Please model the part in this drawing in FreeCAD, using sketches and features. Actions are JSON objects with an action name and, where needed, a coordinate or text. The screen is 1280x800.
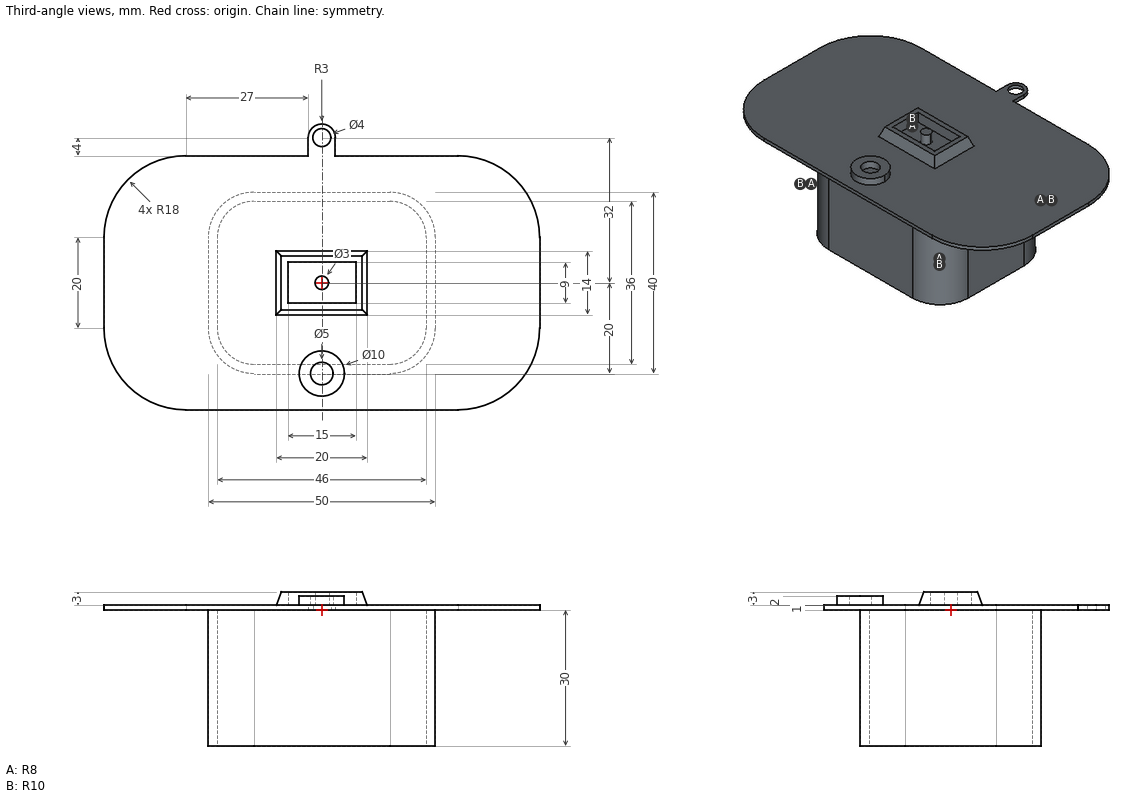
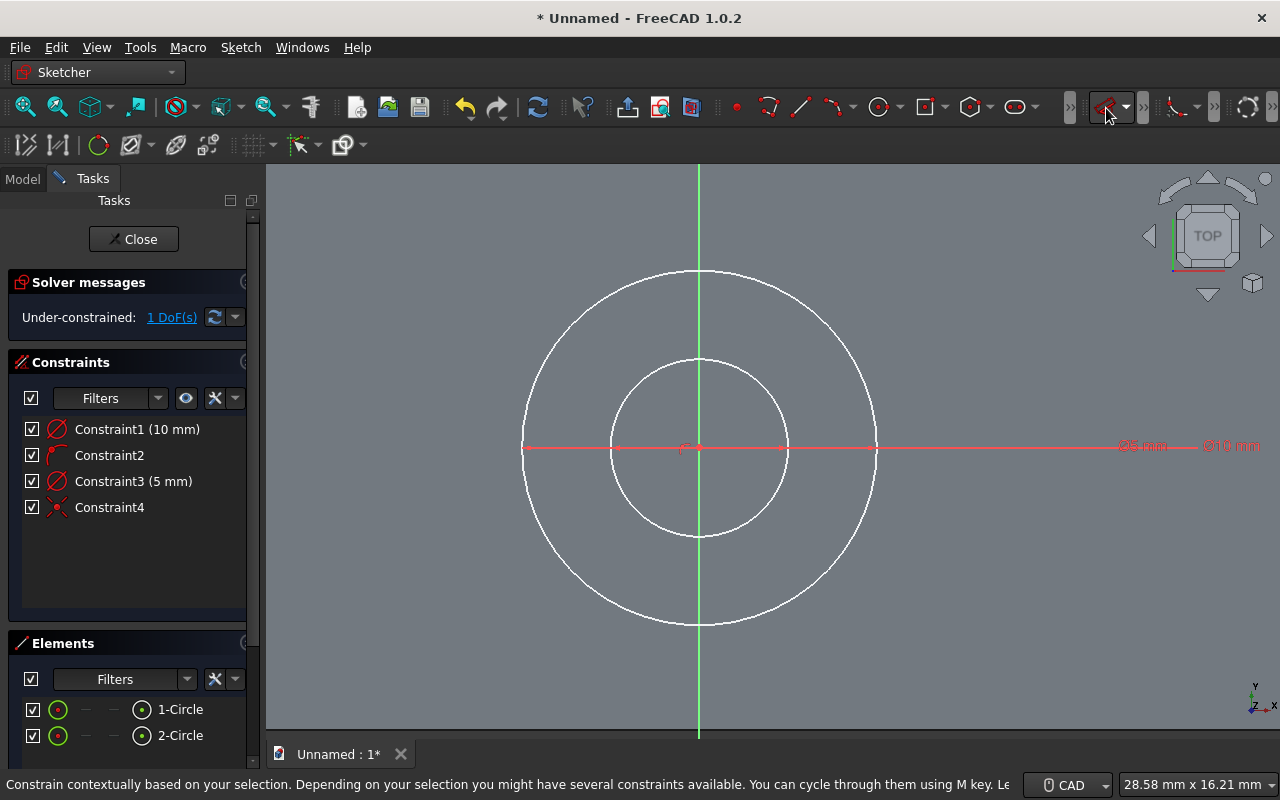
{"action": "left_click", "coordinate": [699, 448]}
{"action": "left_click", "coordinate": [733, 320]}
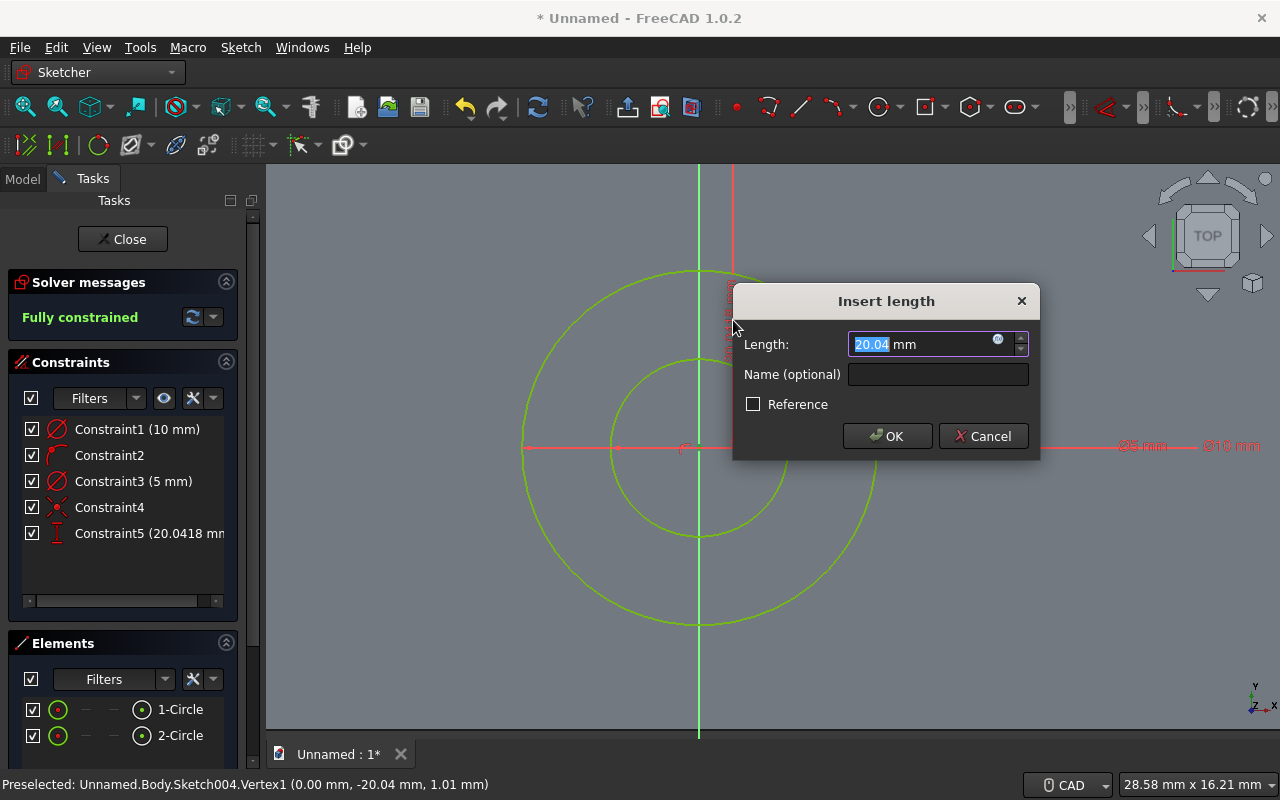
{"action": "type", "text": "20"}
{"action": "key", "text": "Return"}
{"action": "key", "text": "Escape"}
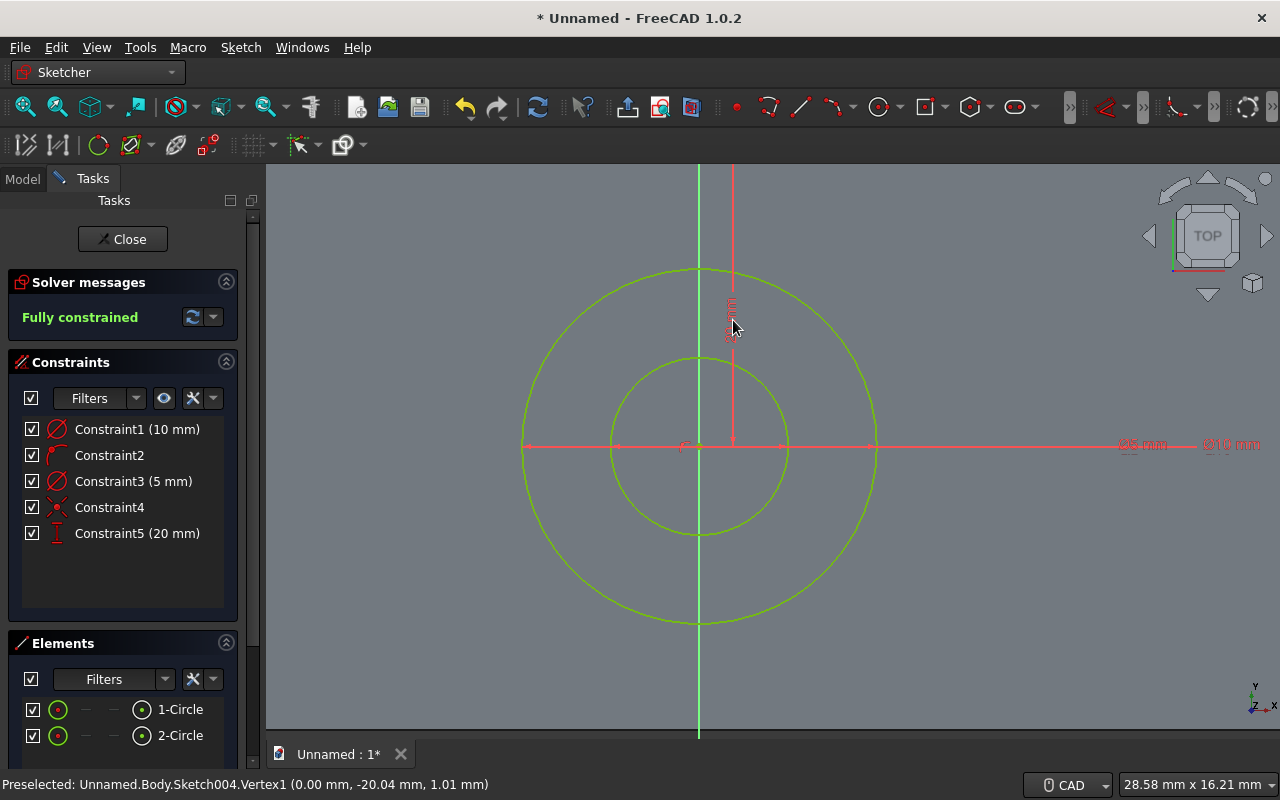
{"action": "left_click", "coordinate": [123, 239]}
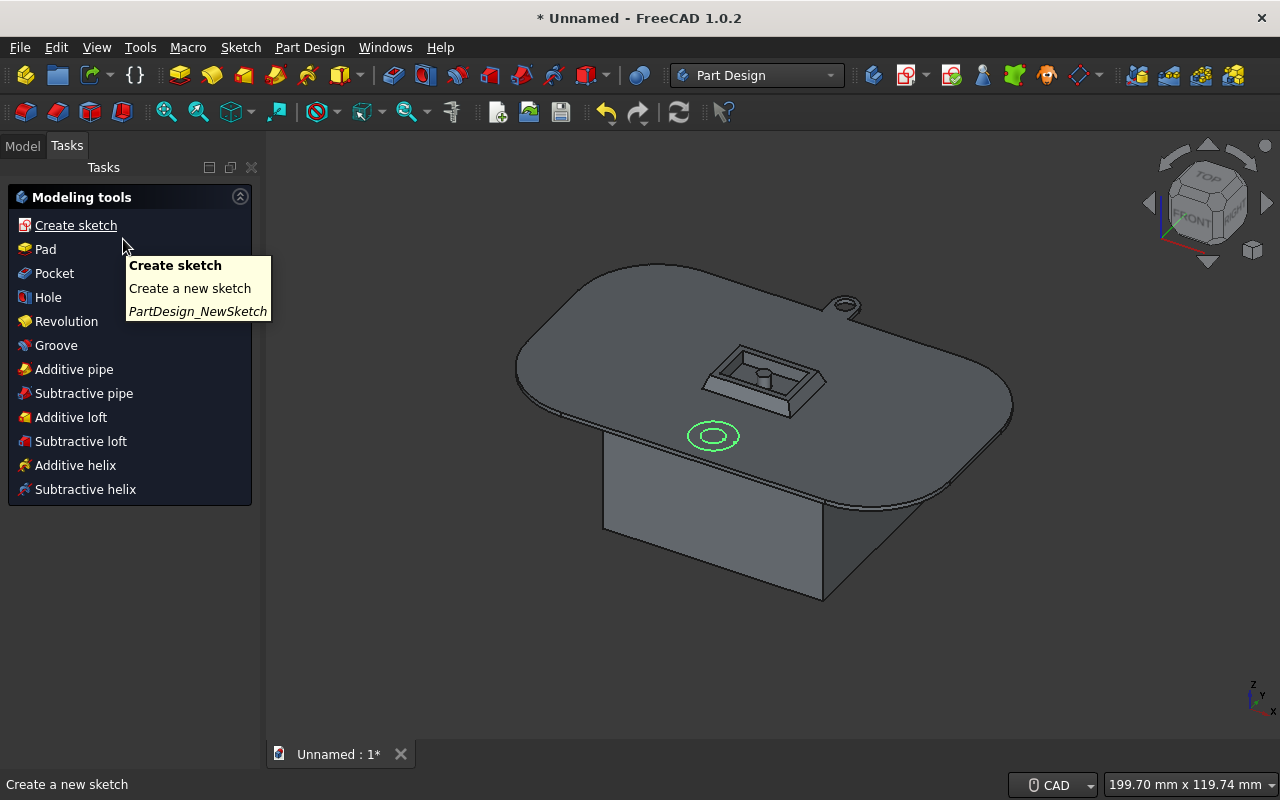
{"action": "left_click", "coordinate": [180, 76]}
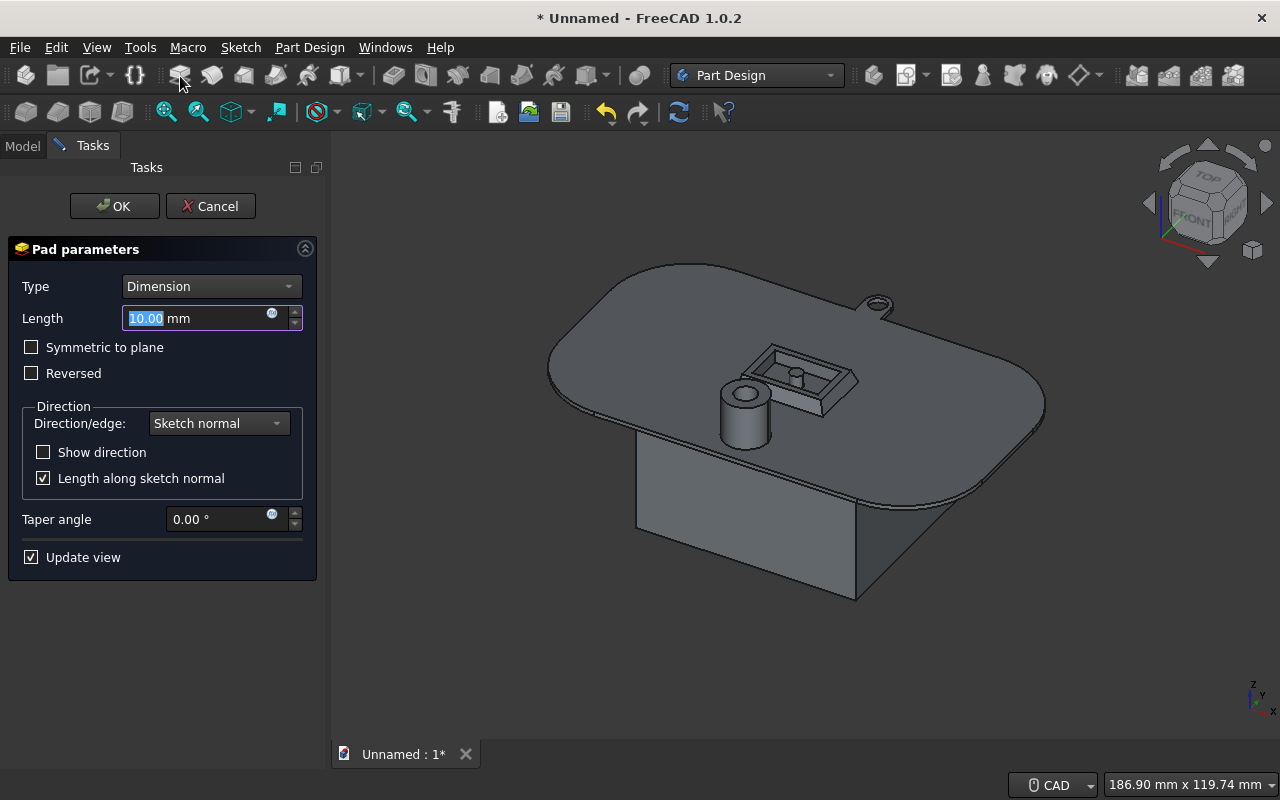
{"action": "type", "text": "2"}
{"action": "key", "text": "Tab"}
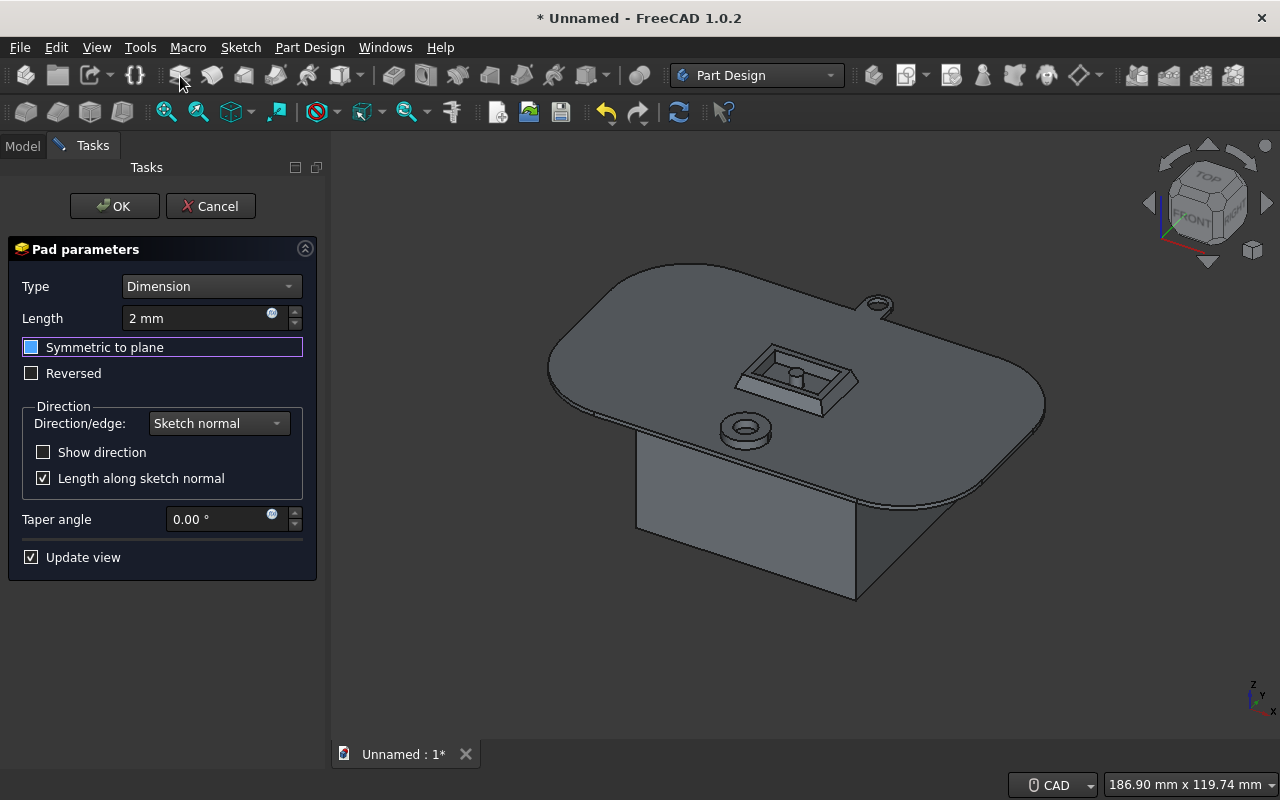
{"action": "left_click", "coordinate": [115, 206]}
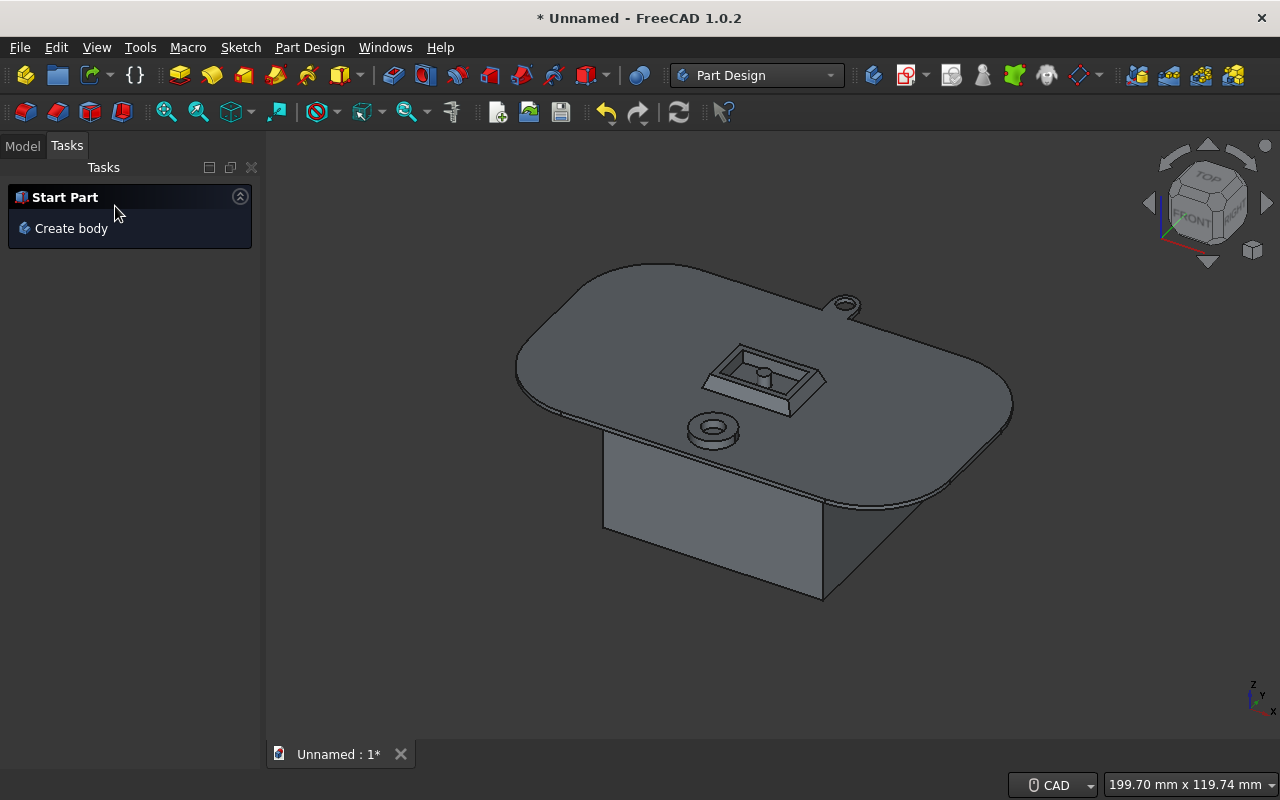
{"action": "key", "text": "0"}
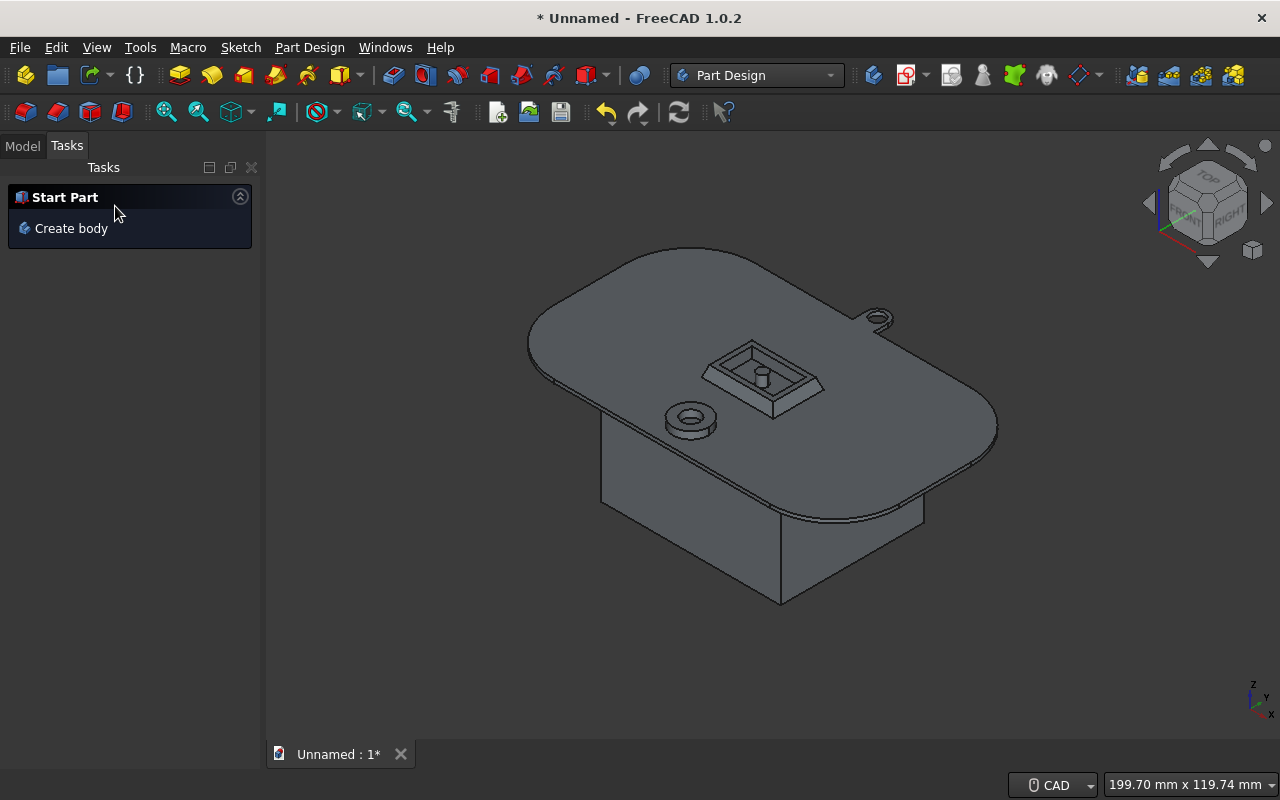
{"action": "key", "text": "2"}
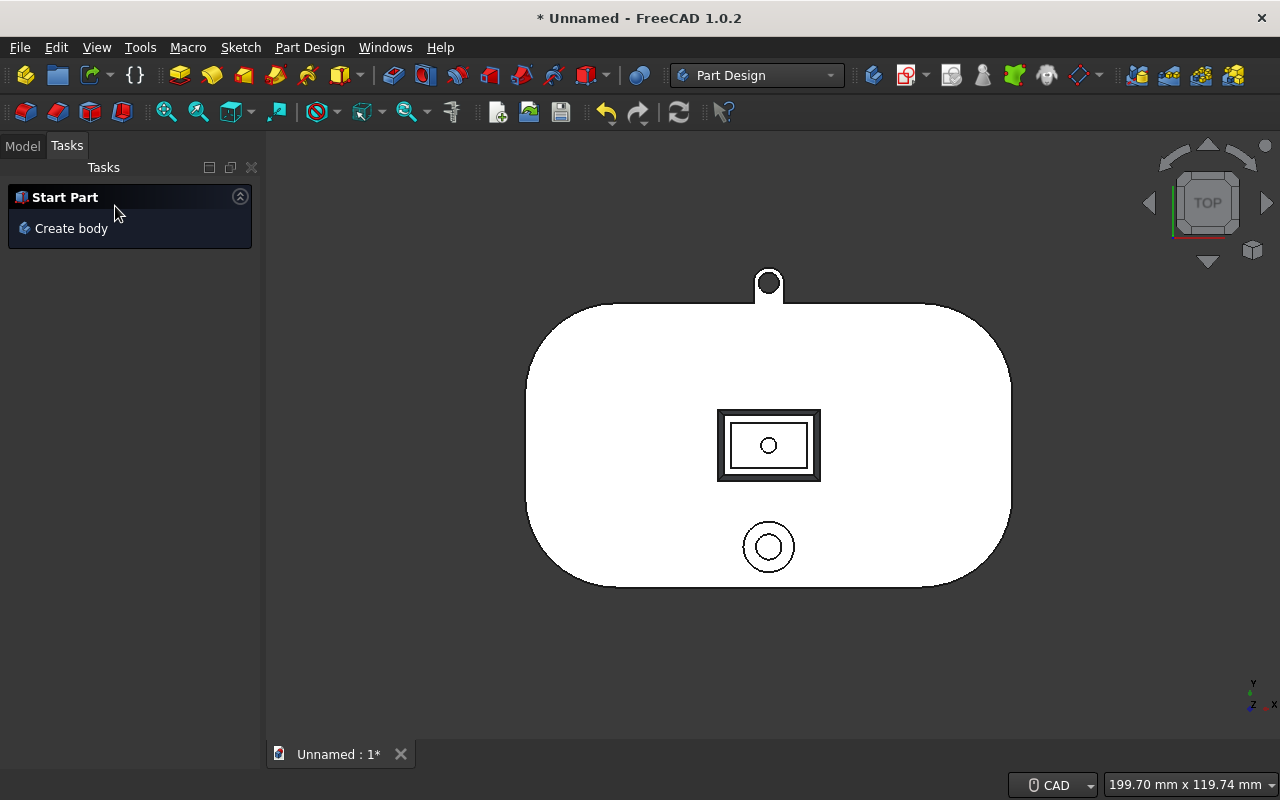
{"action": "key", "text": "1"}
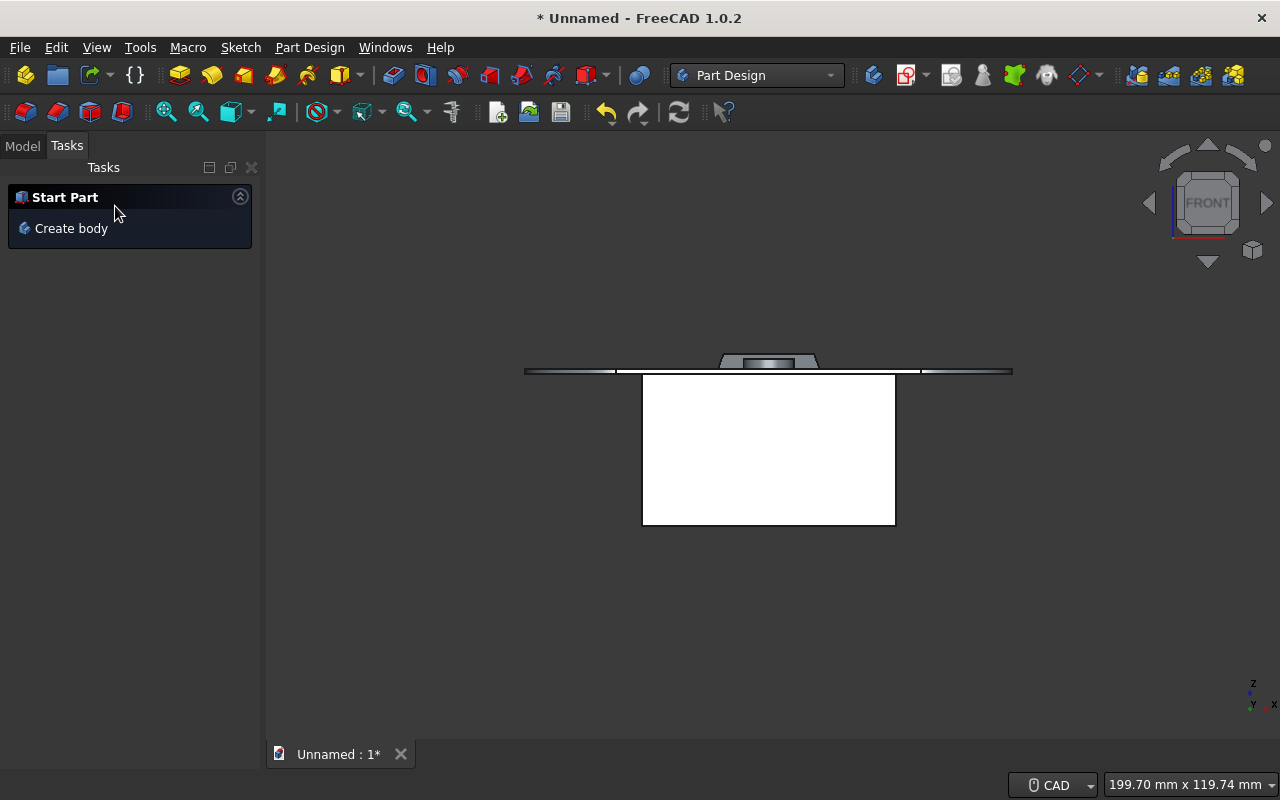
{"action": "key", "text": "3"}